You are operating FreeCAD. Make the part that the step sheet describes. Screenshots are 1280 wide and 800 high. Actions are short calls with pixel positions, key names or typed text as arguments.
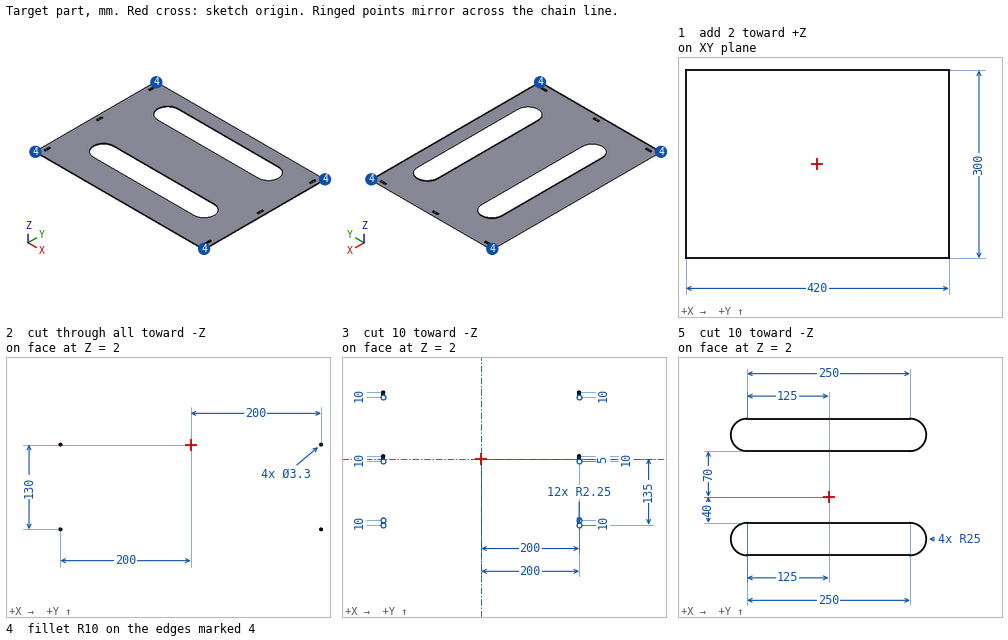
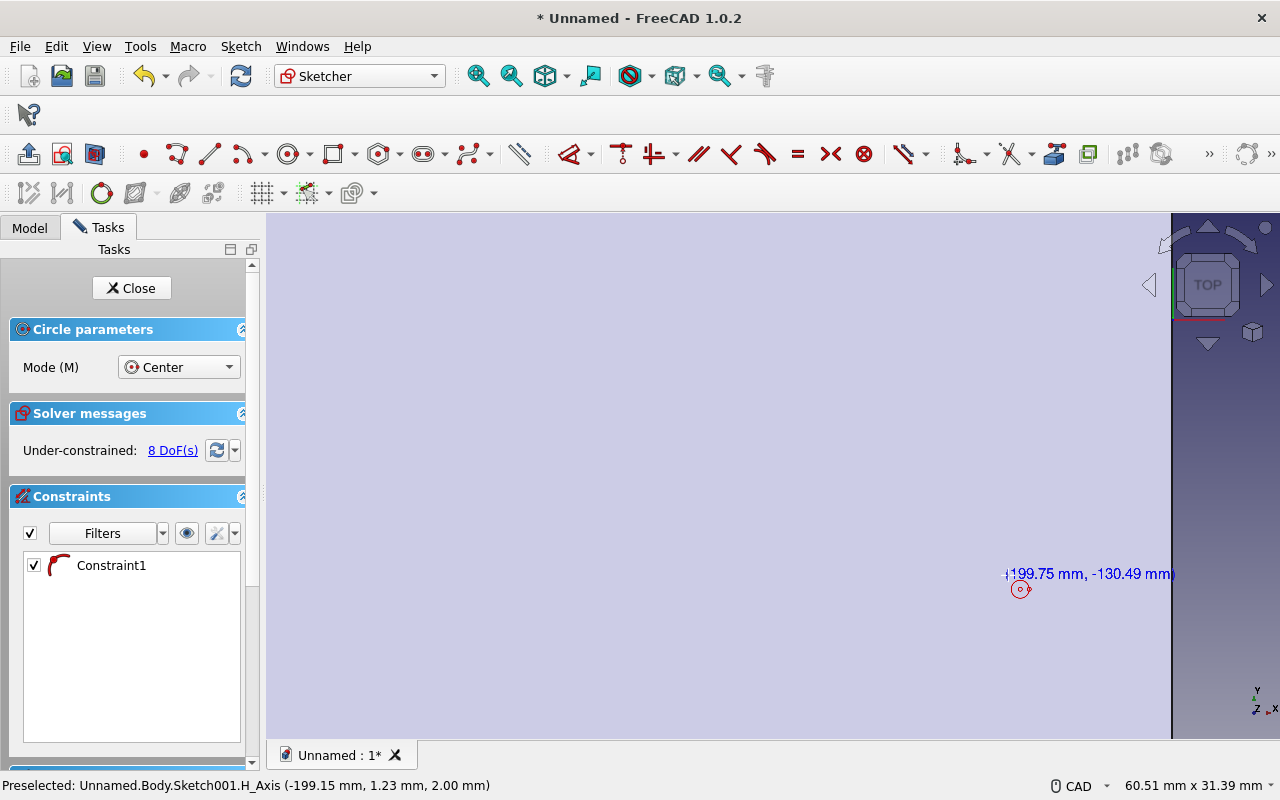
scroll(1009, 575, down, 12)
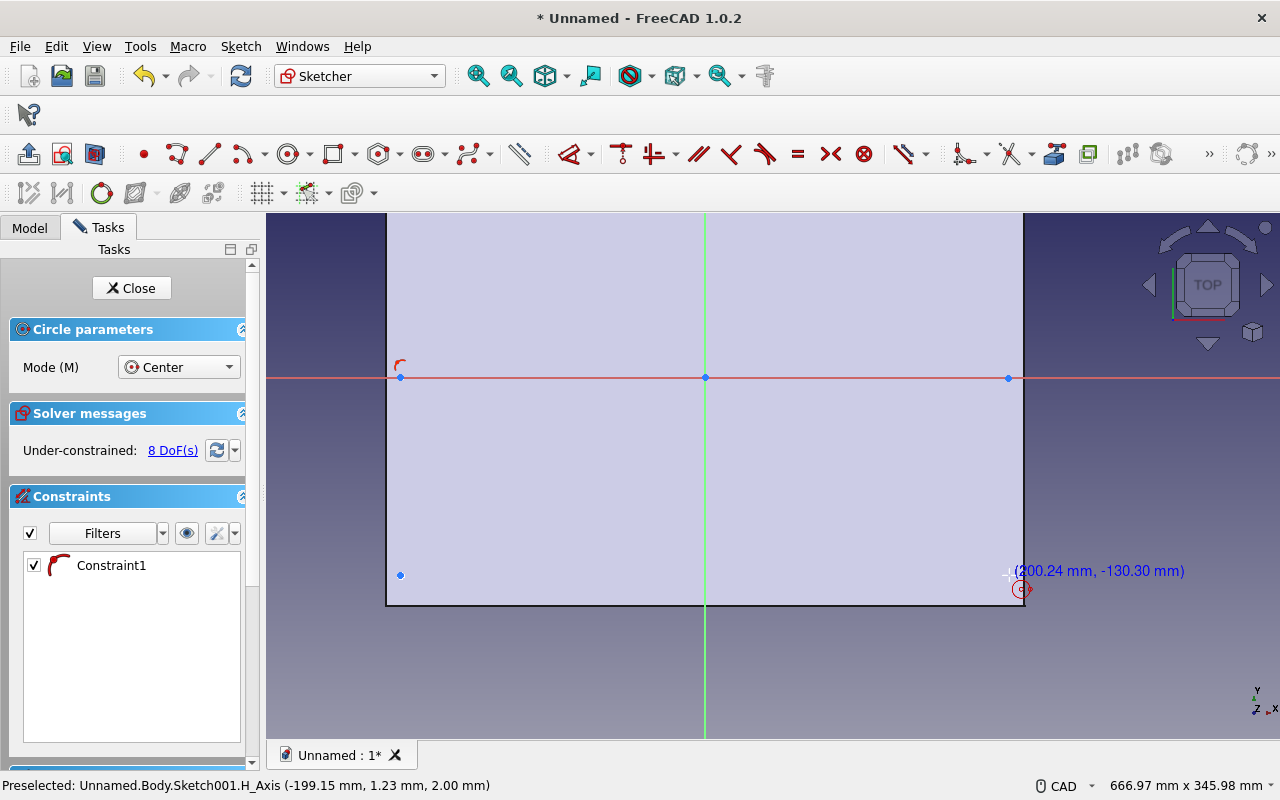
click(1009, 575)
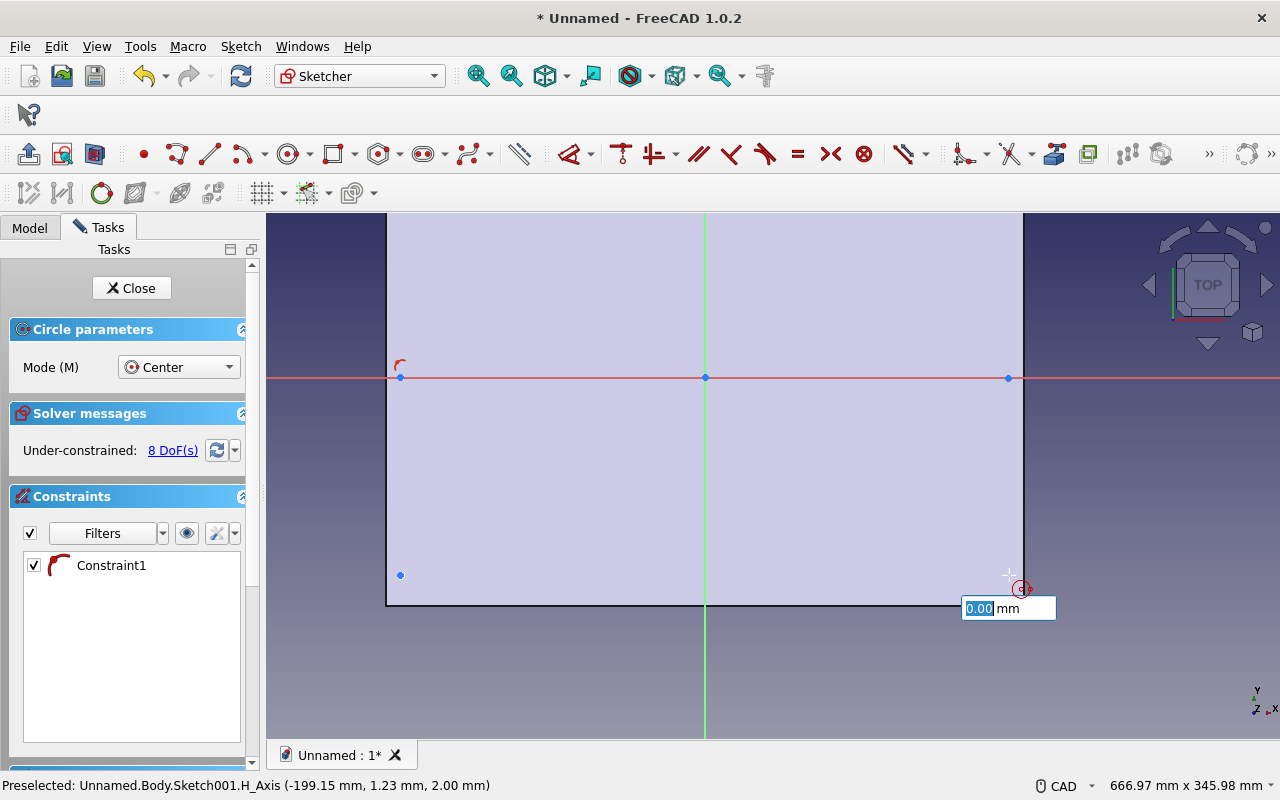
scroll(1011, 573, up, 10)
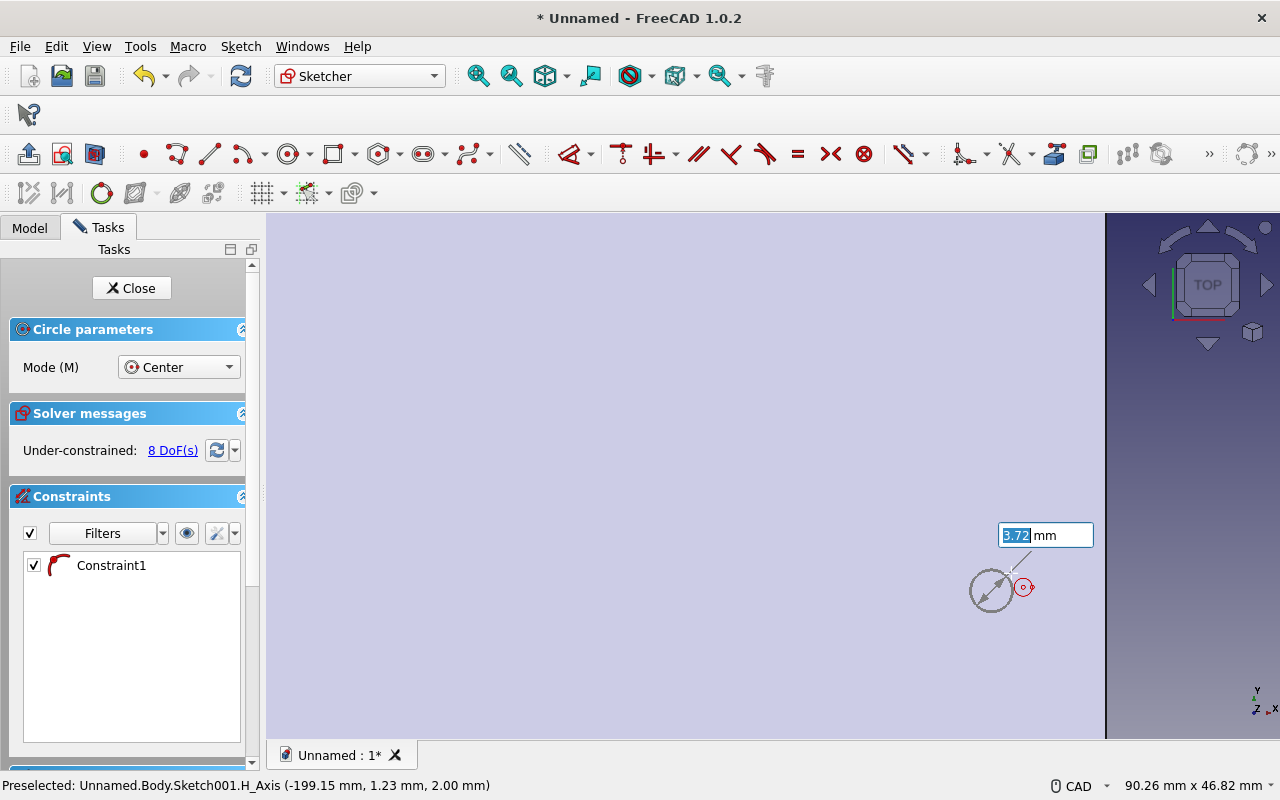
click(1007, 572)
key(Escape)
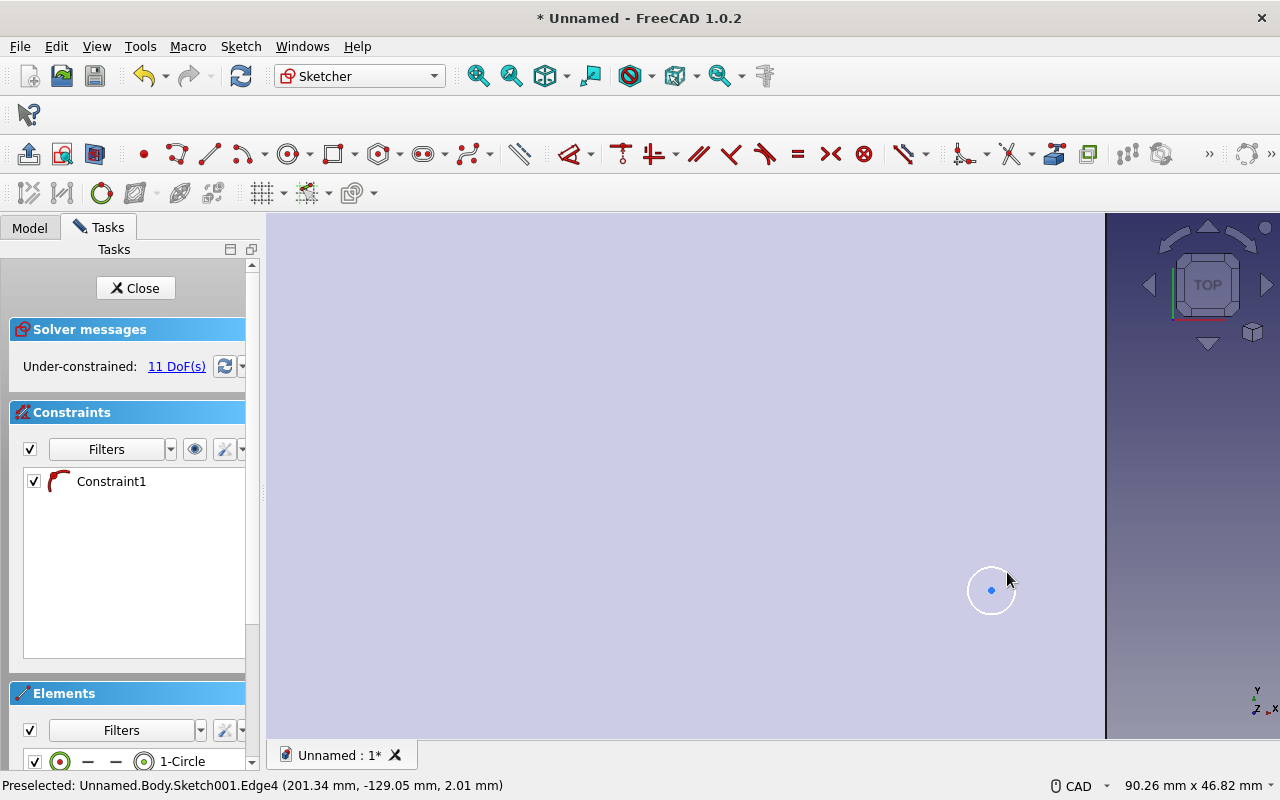
scroll(1011, 573, down, 10)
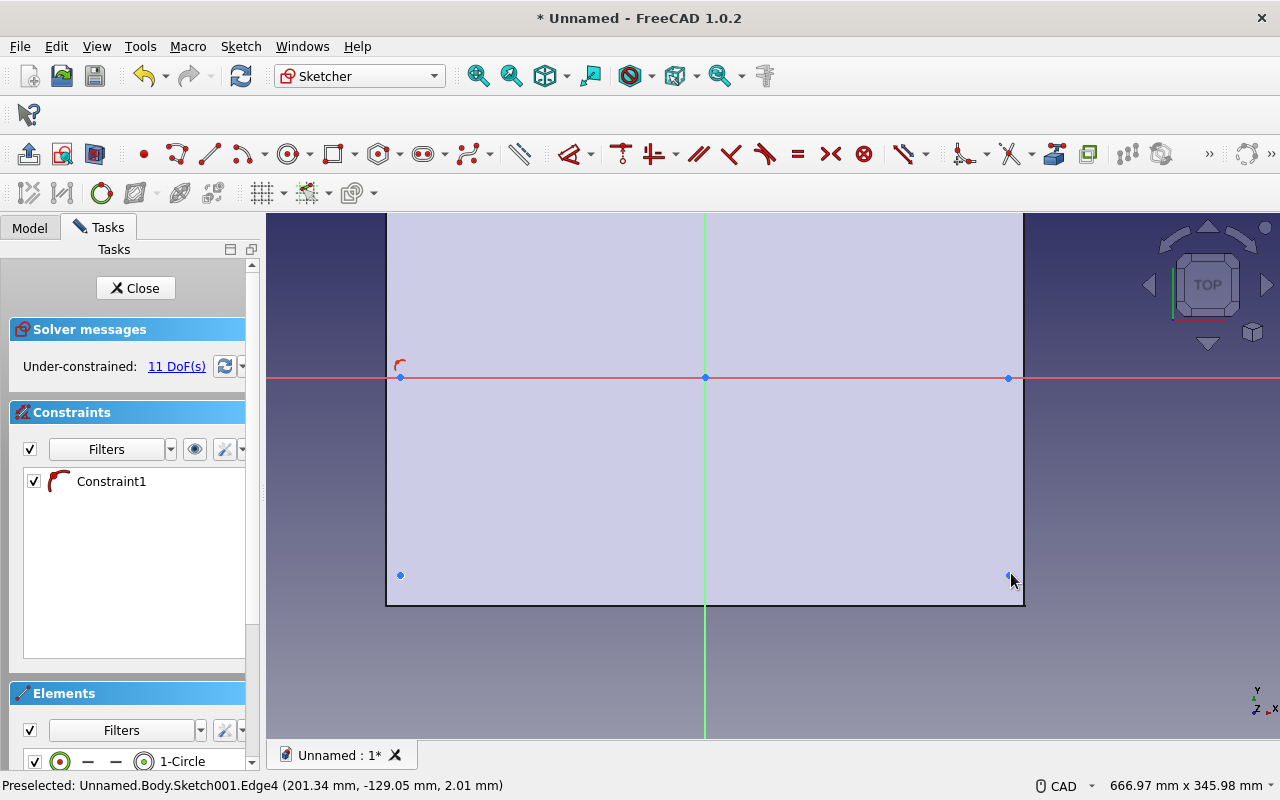
scroll(1010, 378, up, 13)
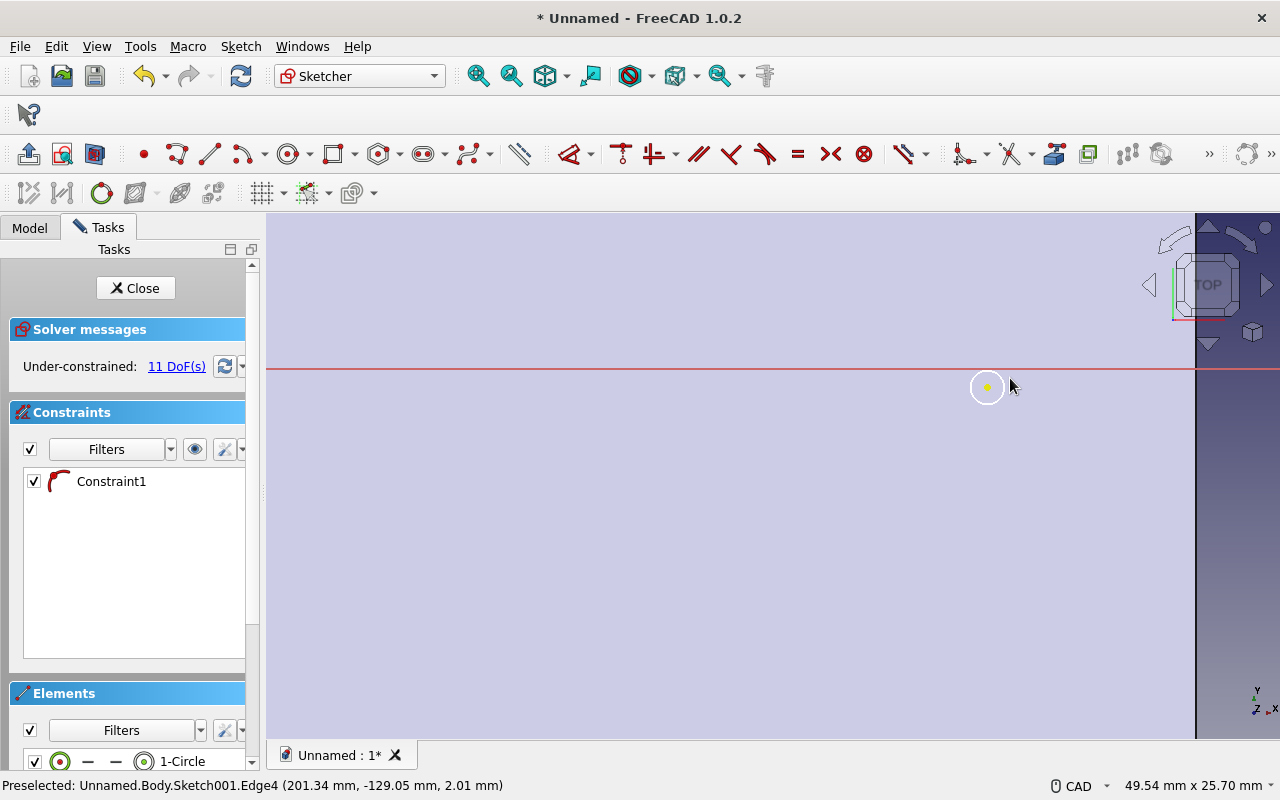
click(999, 376)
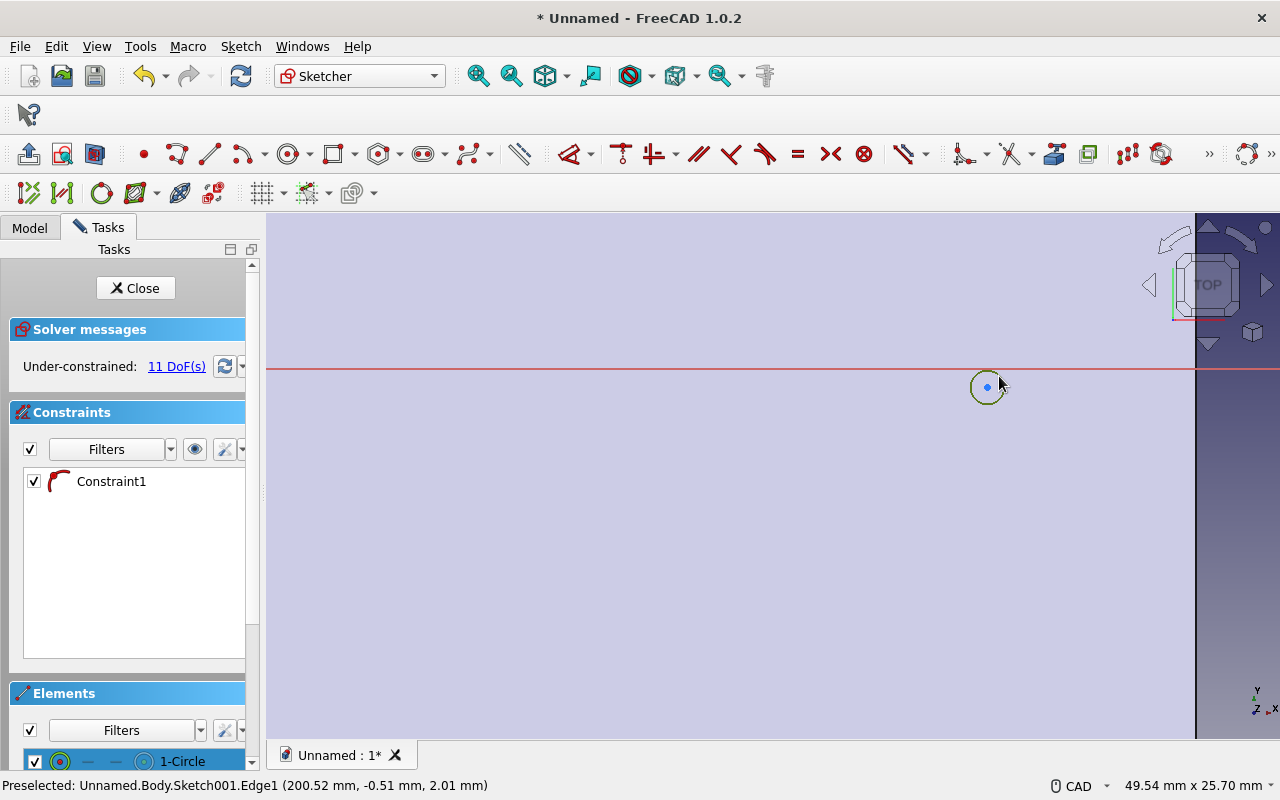
scroll(1010, 378, down, 13)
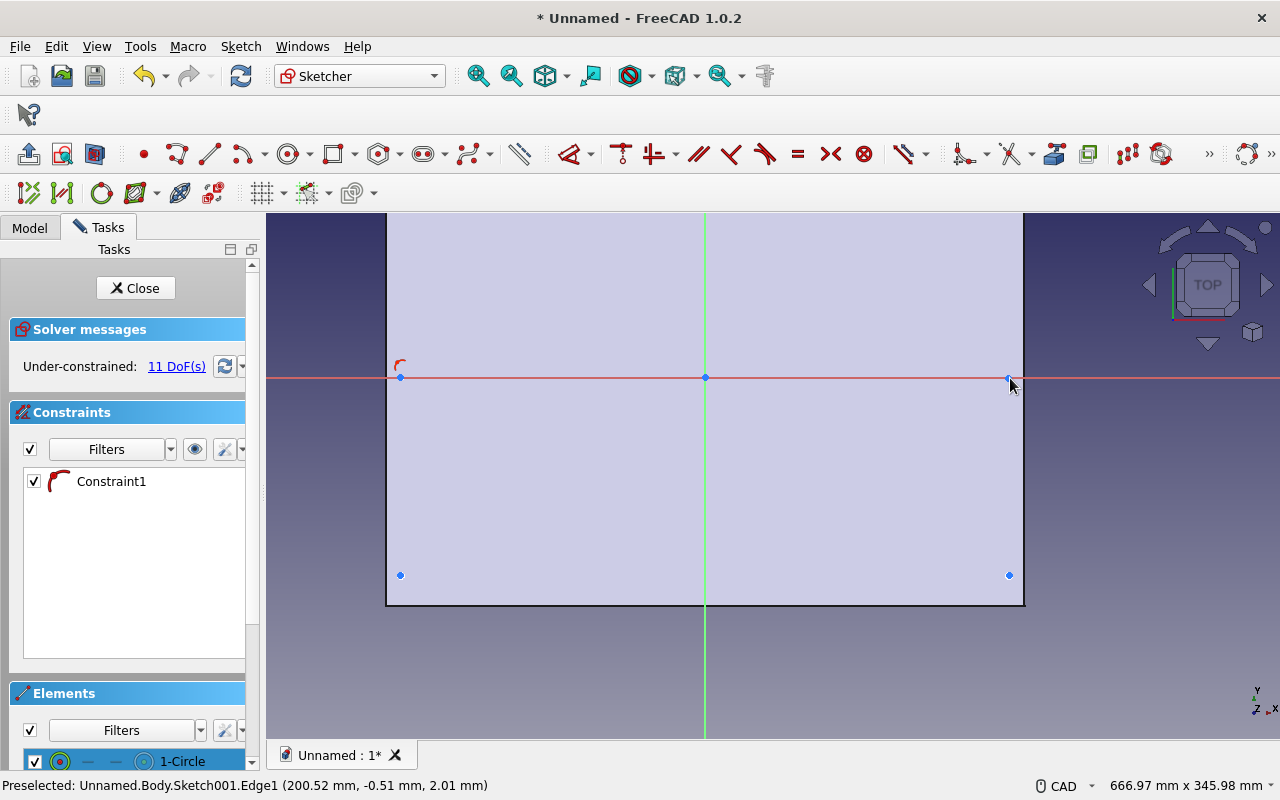
scroll(403, 574, up, 8)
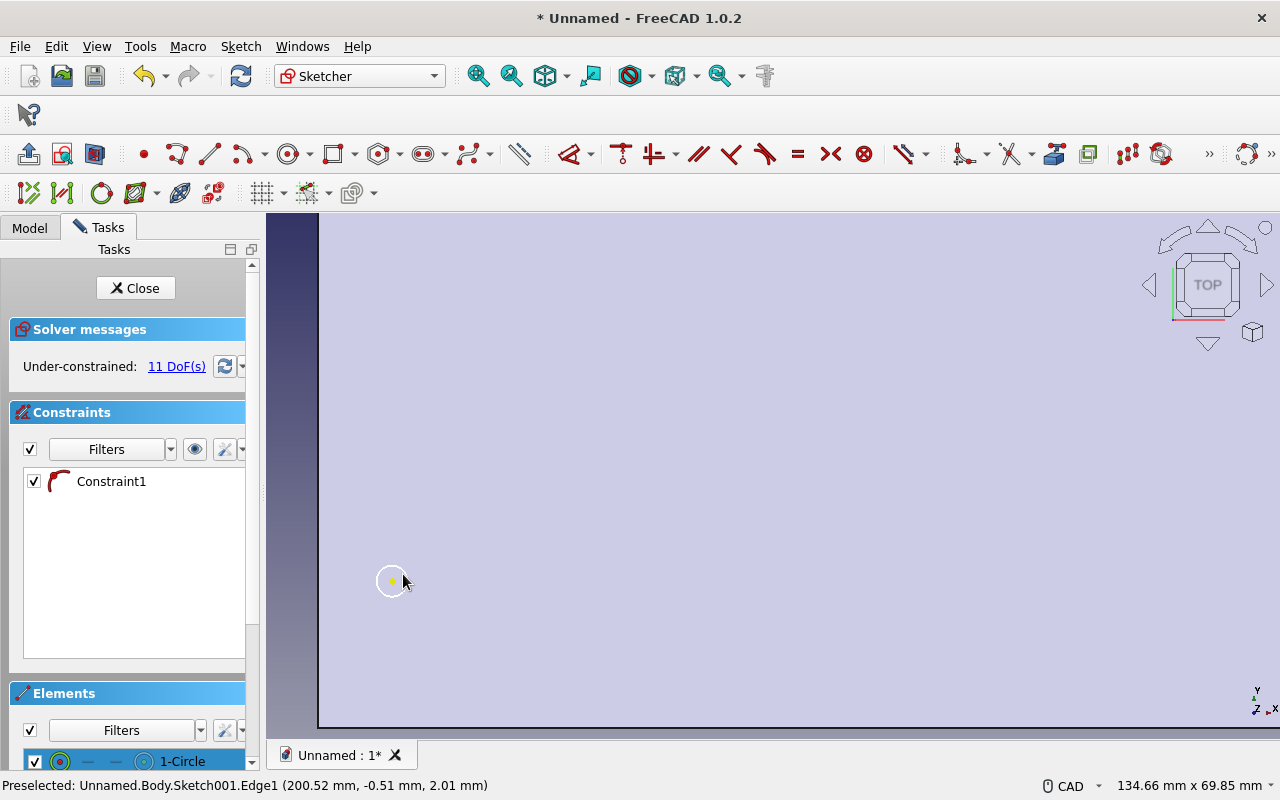
click(403, 570)